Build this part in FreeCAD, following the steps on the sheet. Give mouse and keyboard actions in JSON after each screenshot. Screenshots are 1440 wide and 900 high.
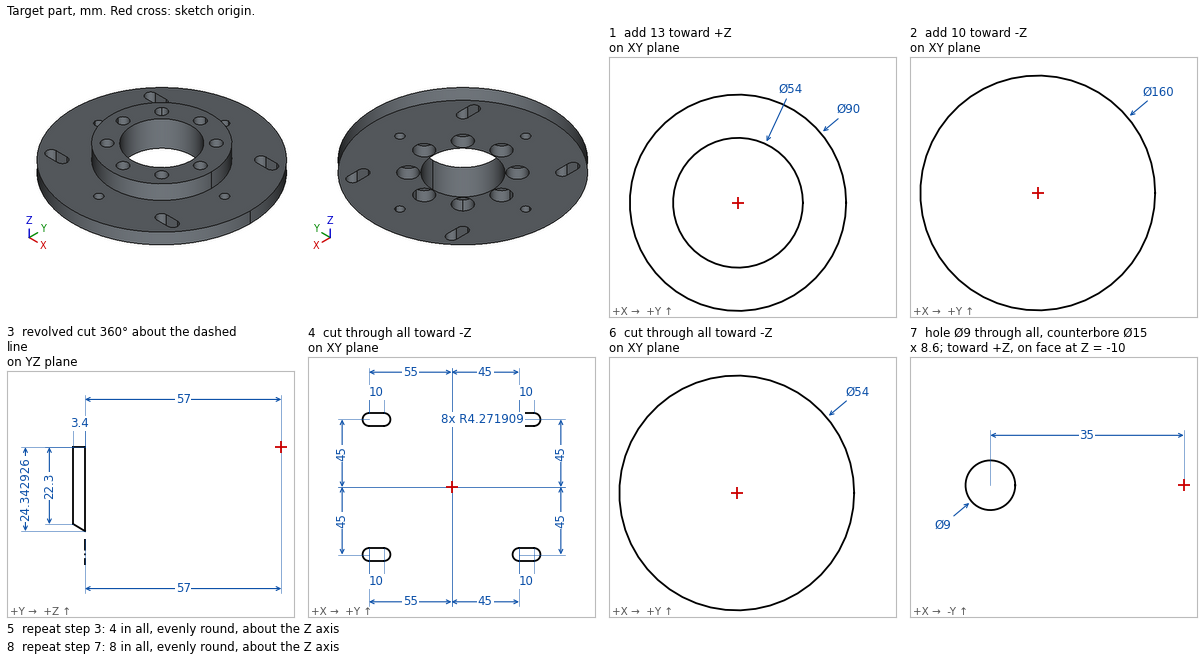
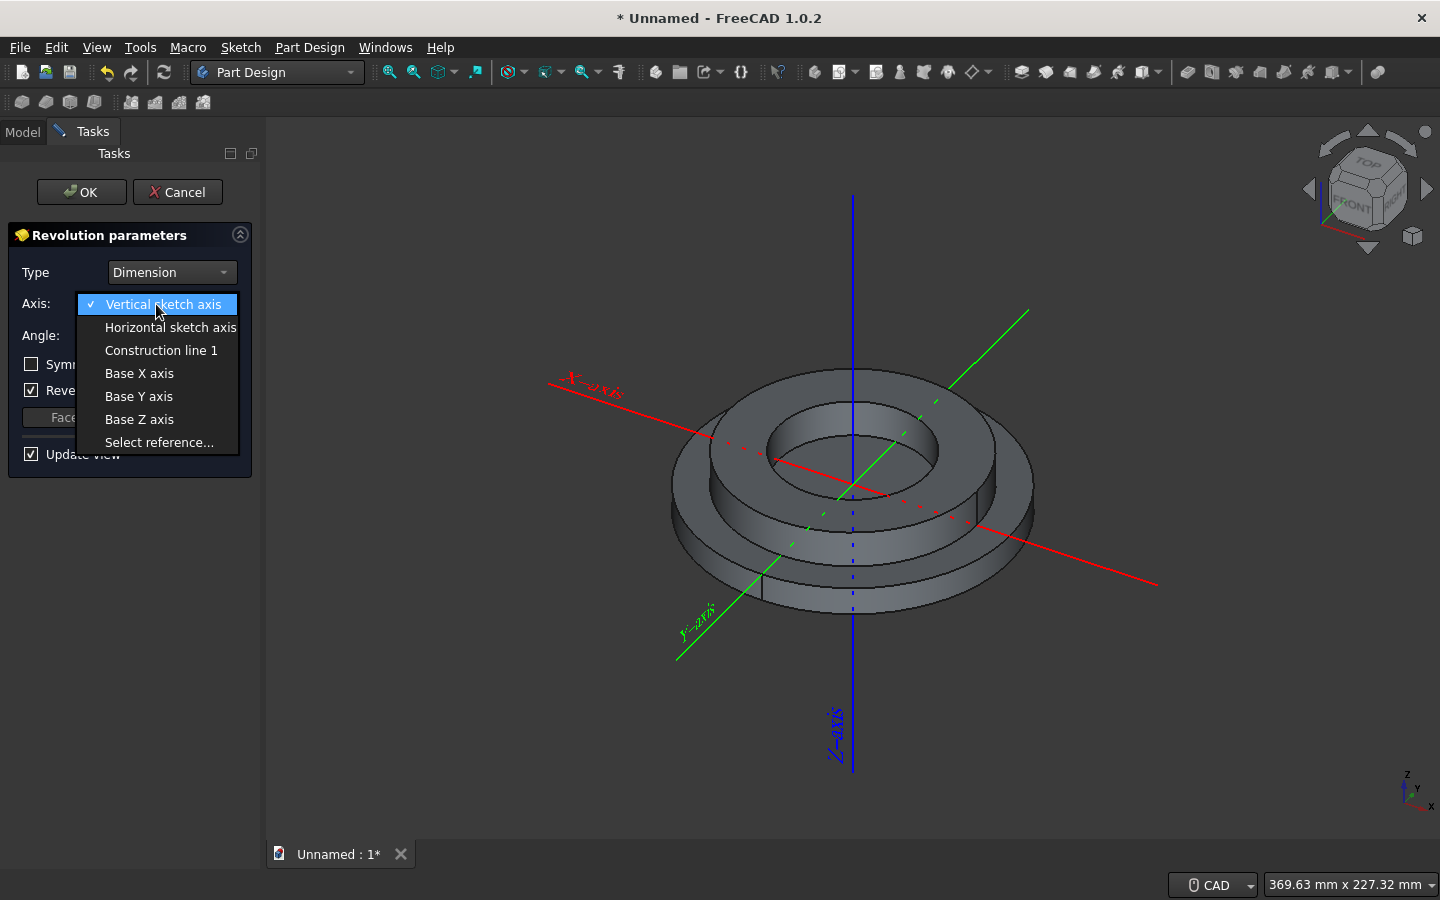
{"action": "left_click", "coordinate": [156, 350]}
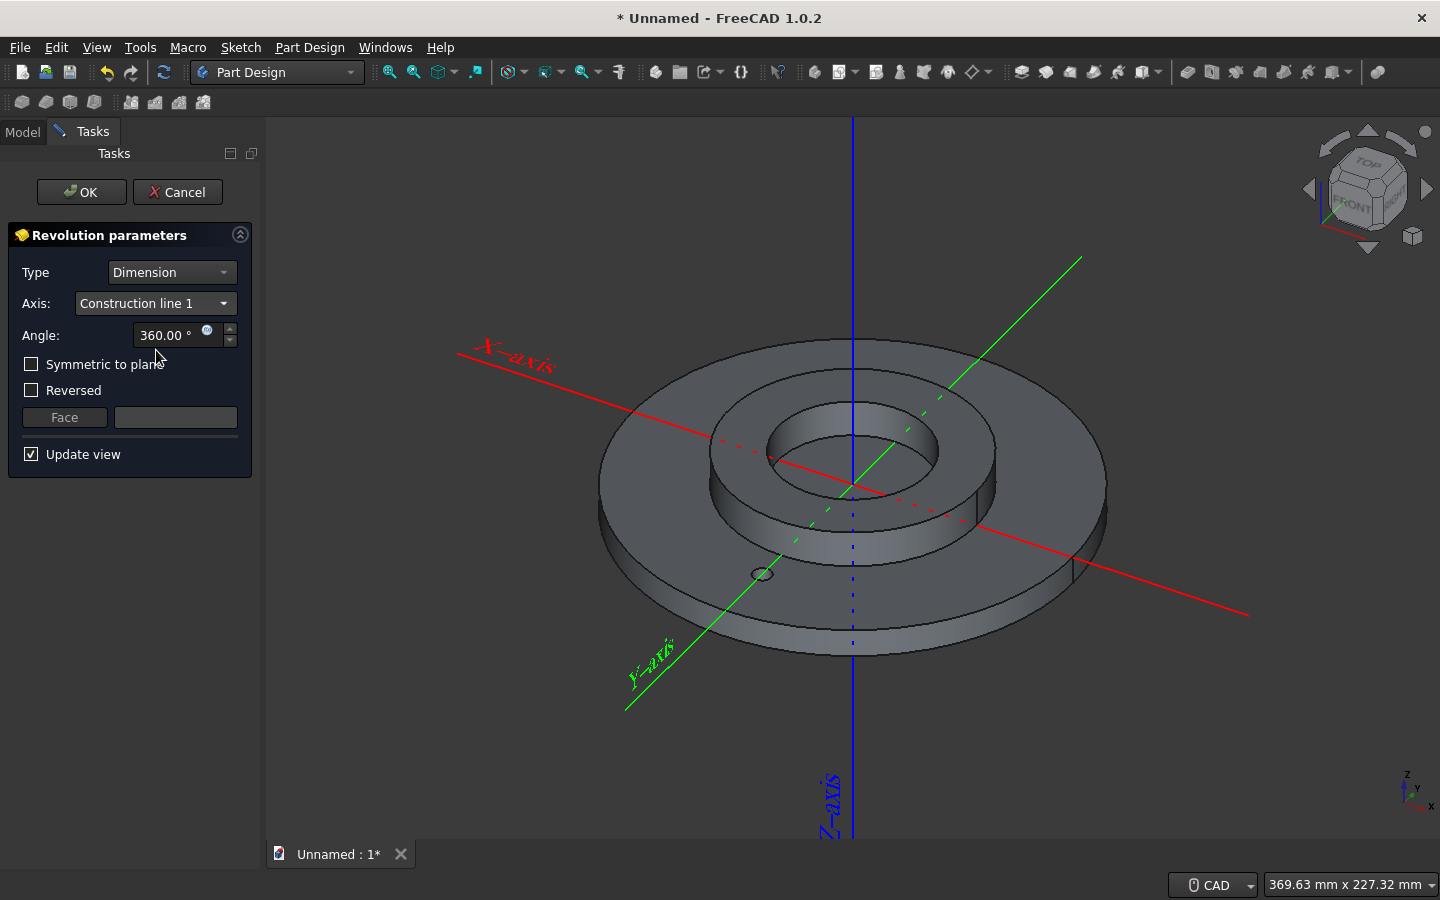
{"action": "left_click", "coordinate": [82, 192]}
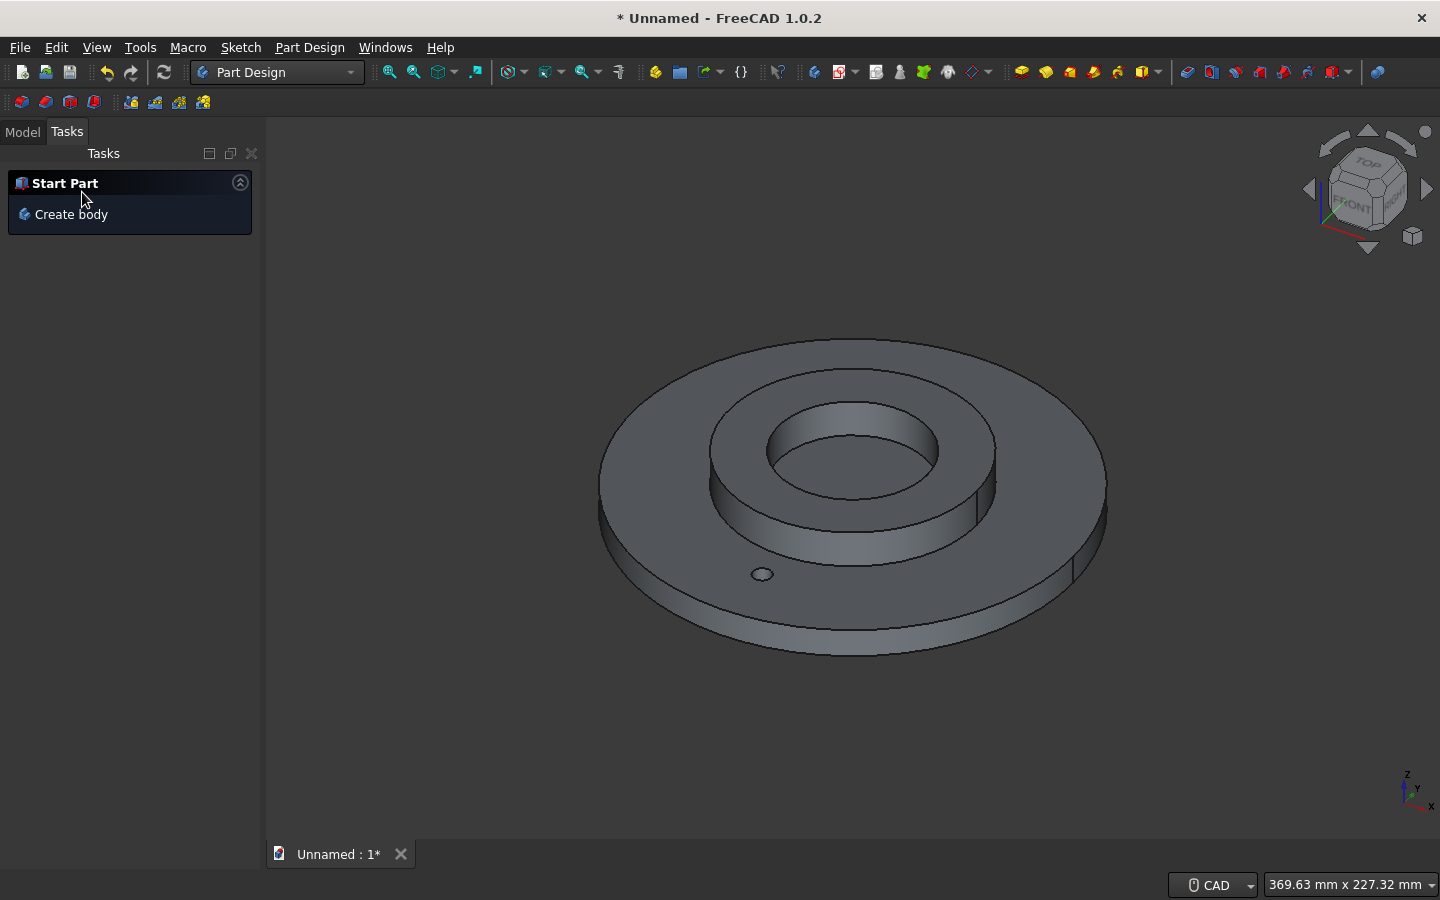
{"action": "left_click", "coordinate": [840, 72]}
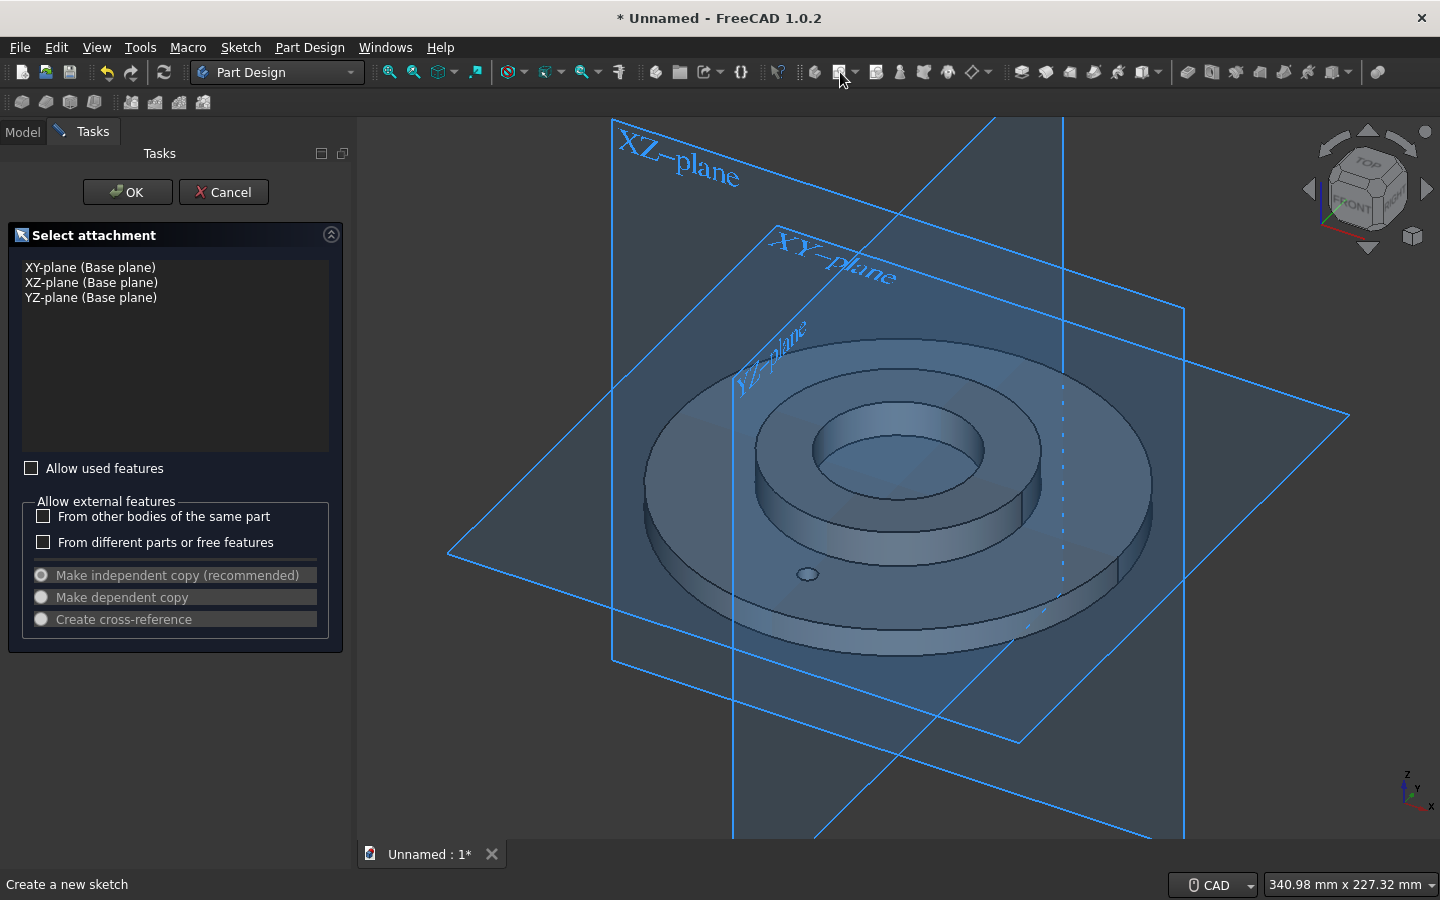
{"action": "left_click", "coordinate": [82, 268]}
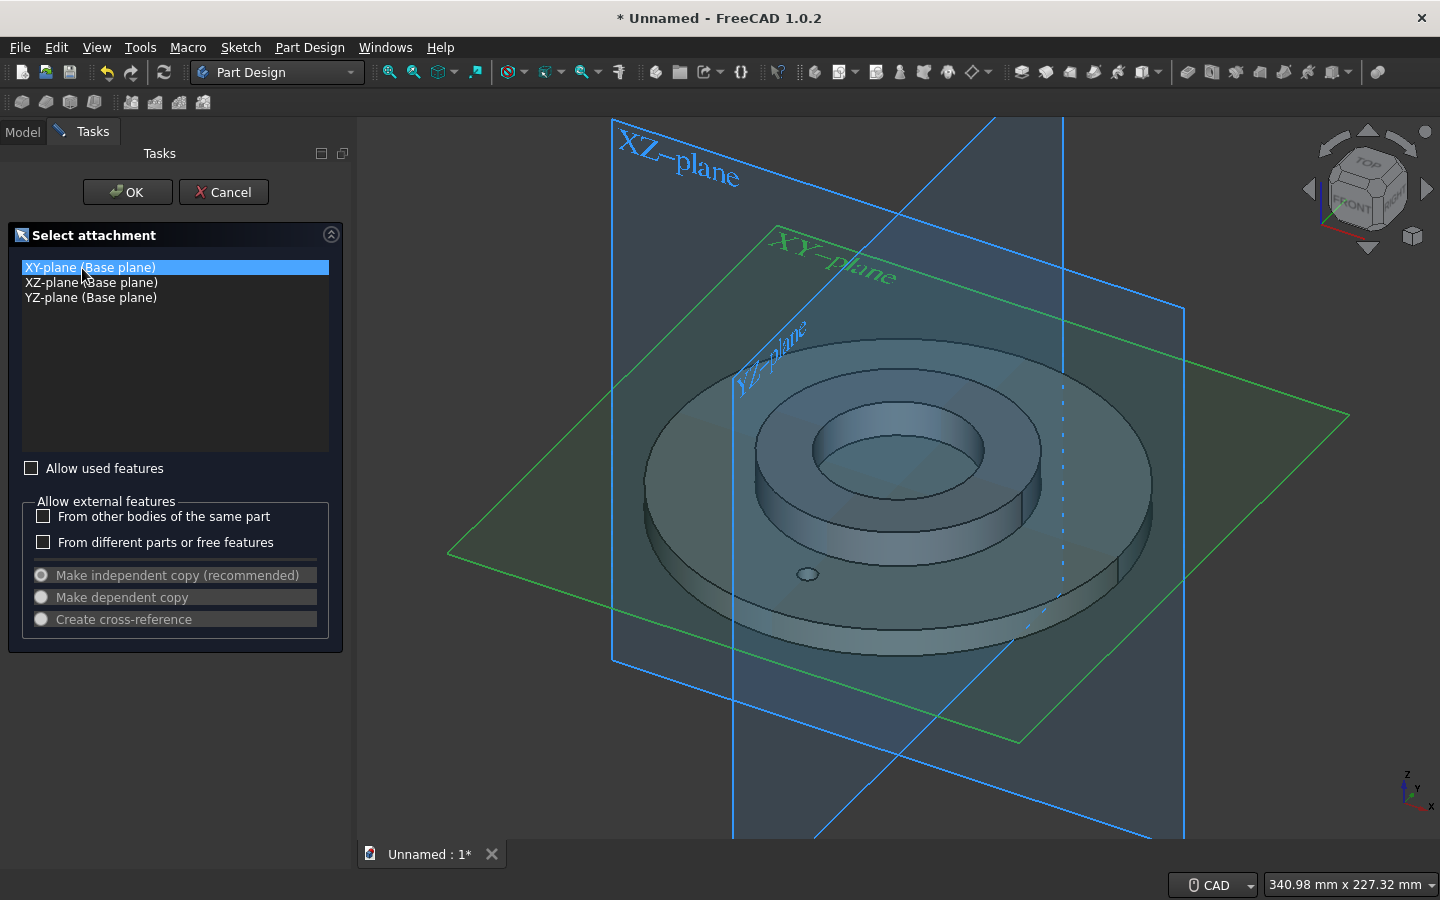
{"action": "left_click", "coordinate": [128, 192]}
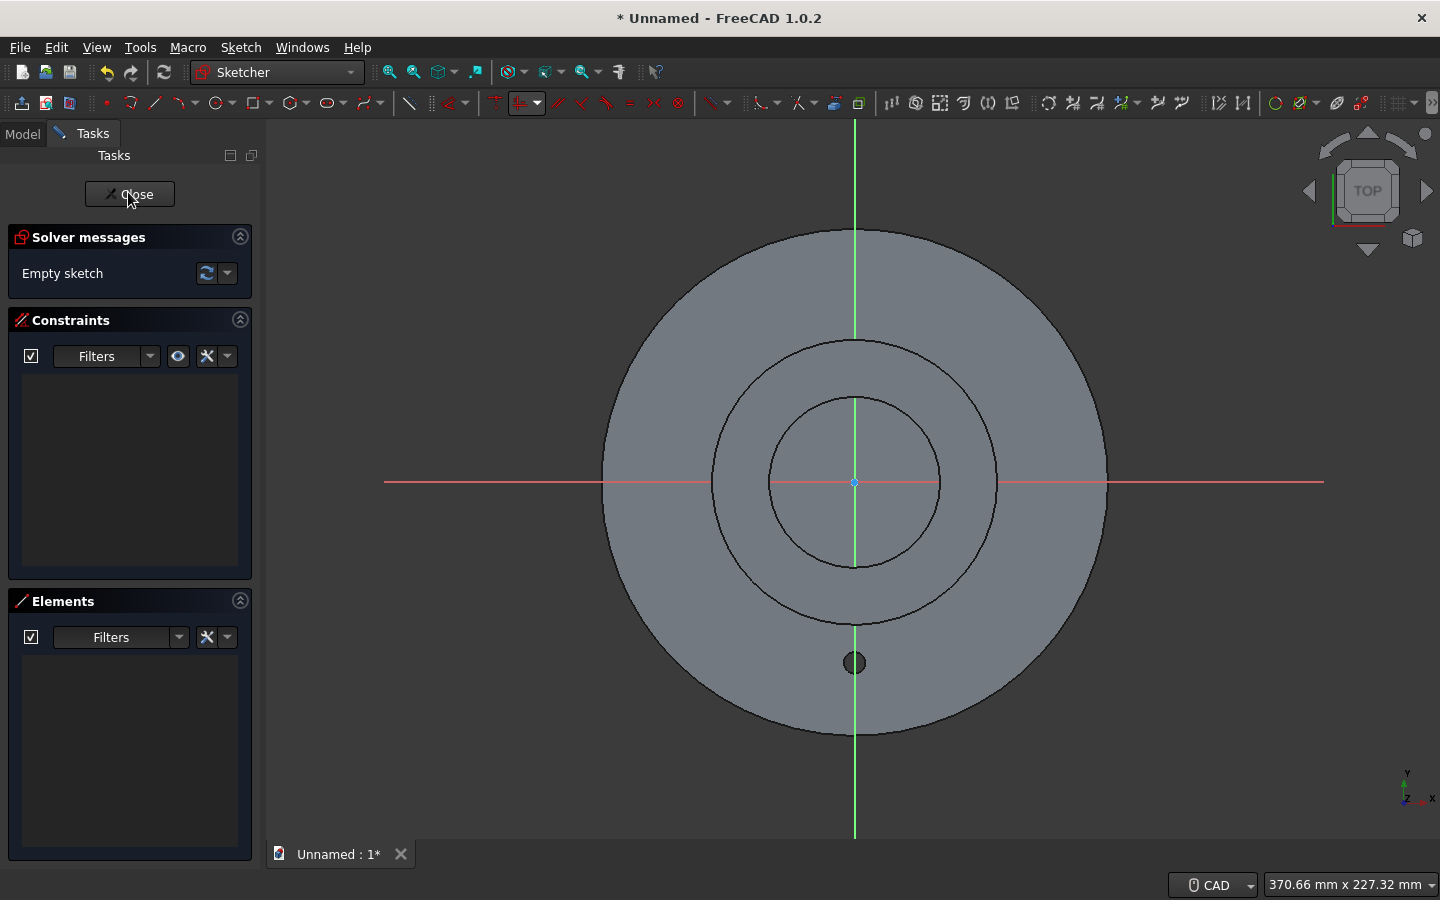
{"action": "left_click", "coordinate": [70, 104]}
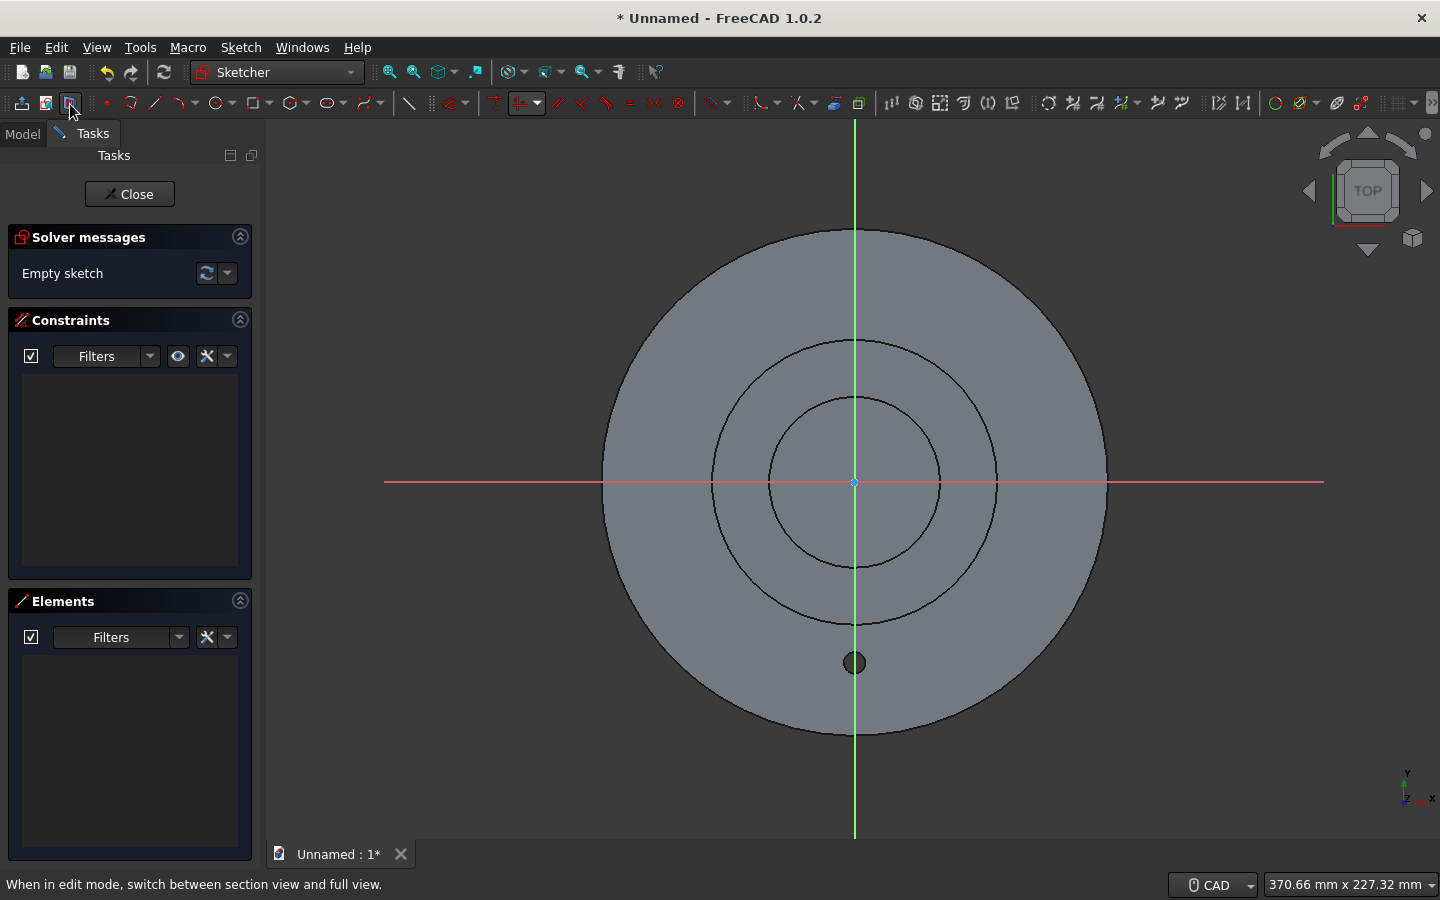
{"action": "scroll", "coordinate": [997, 489], "scroll_direction": "up", "scroll_amount": 2}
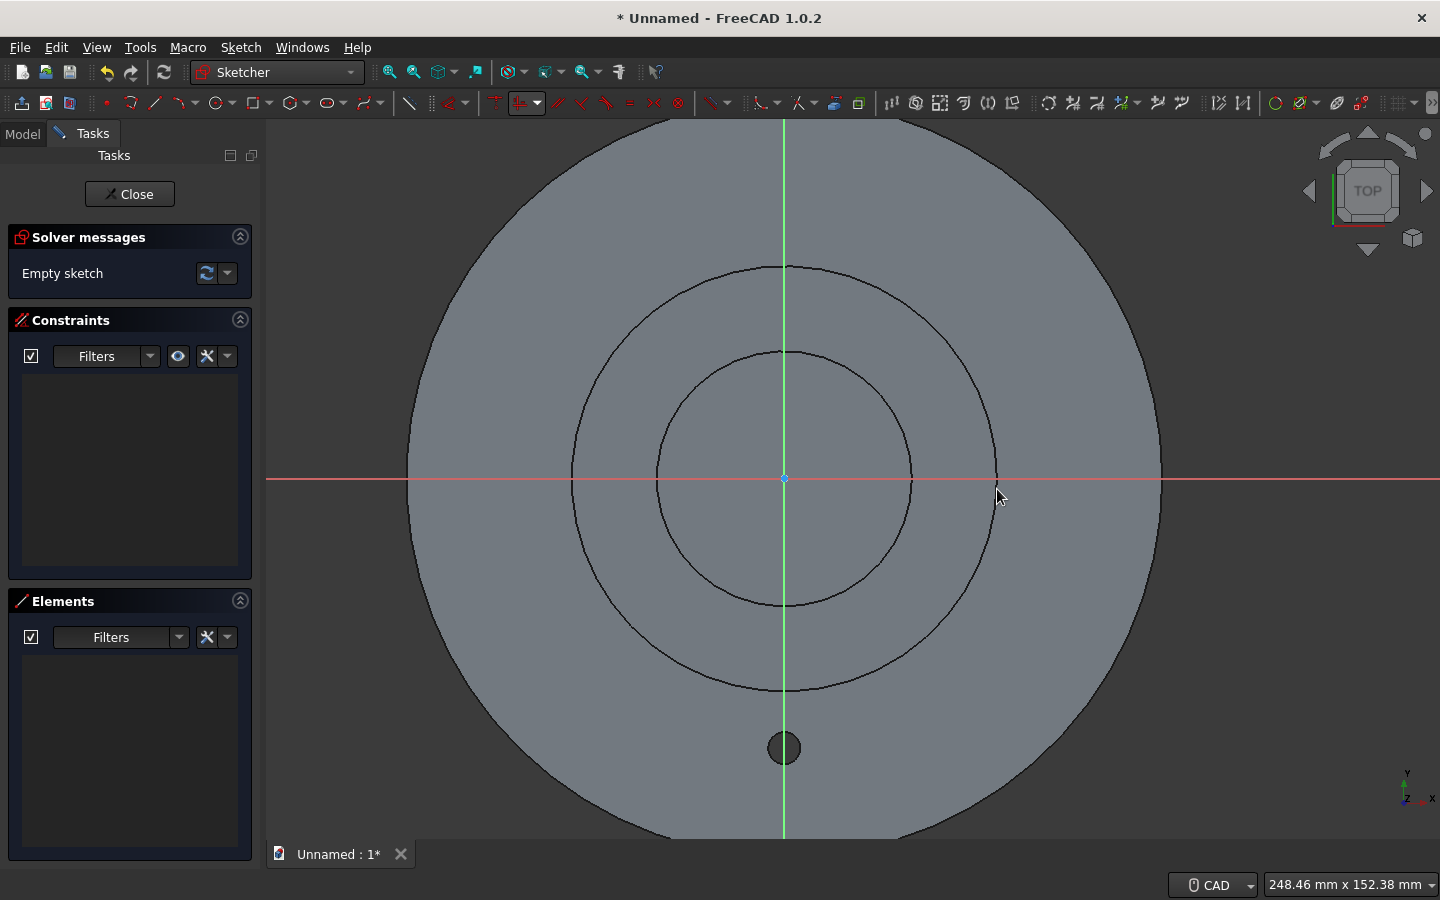
{"action": "key", "text": "g s"}